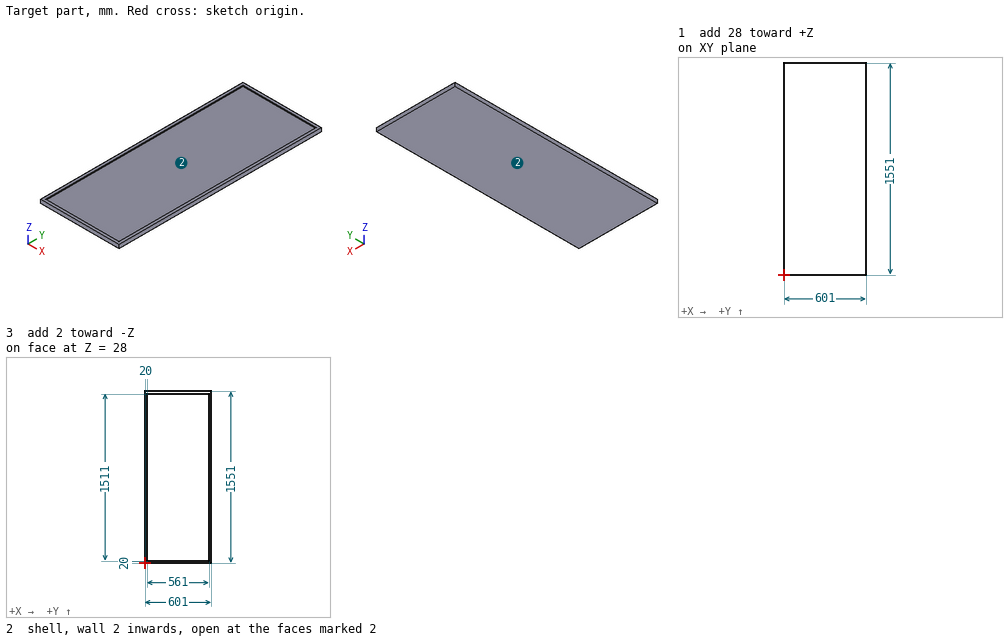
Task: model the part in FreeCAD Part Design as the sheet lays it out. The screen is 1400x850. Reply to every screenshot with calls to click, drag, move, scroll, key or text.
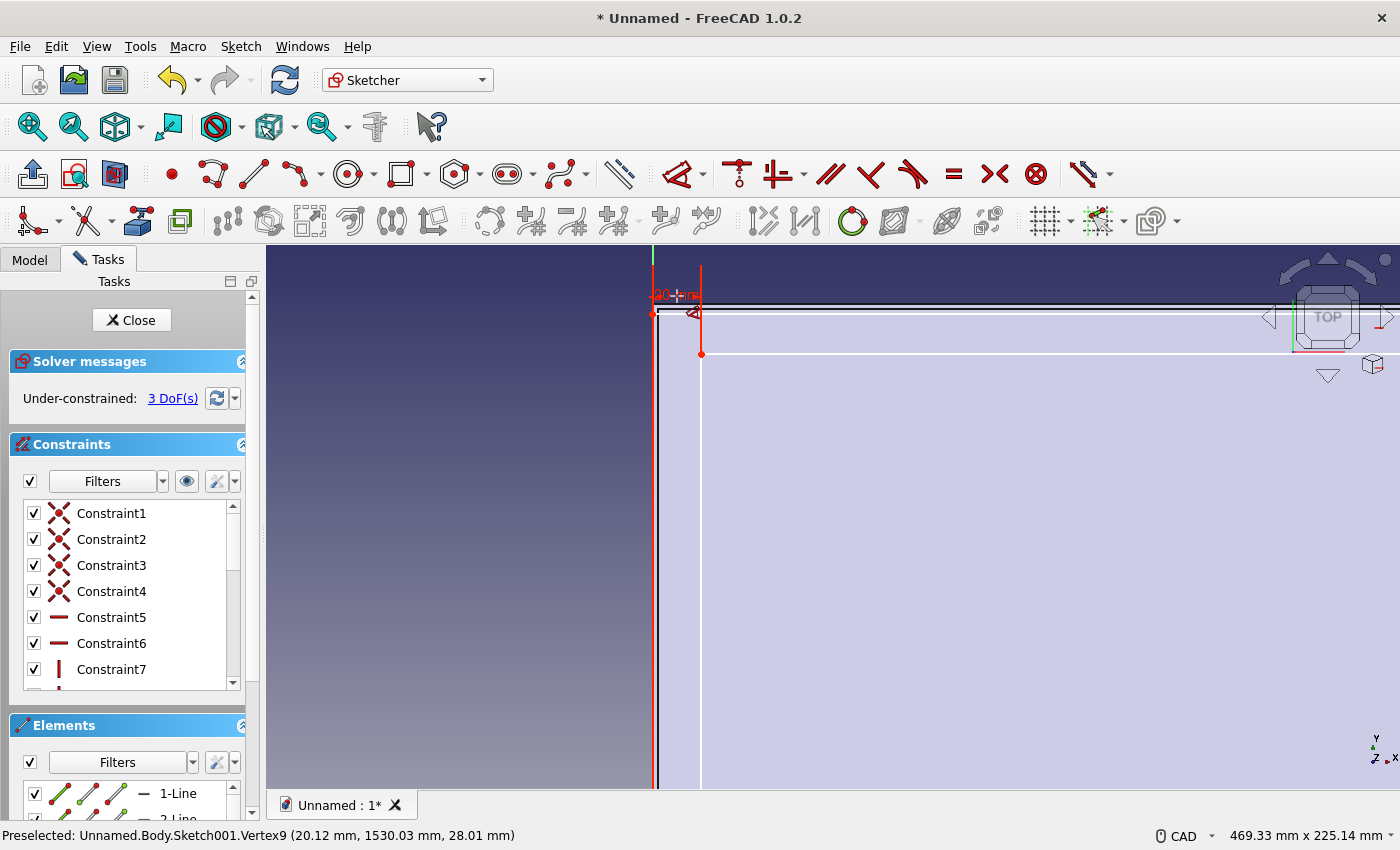
scroll(703, 351, down, 12)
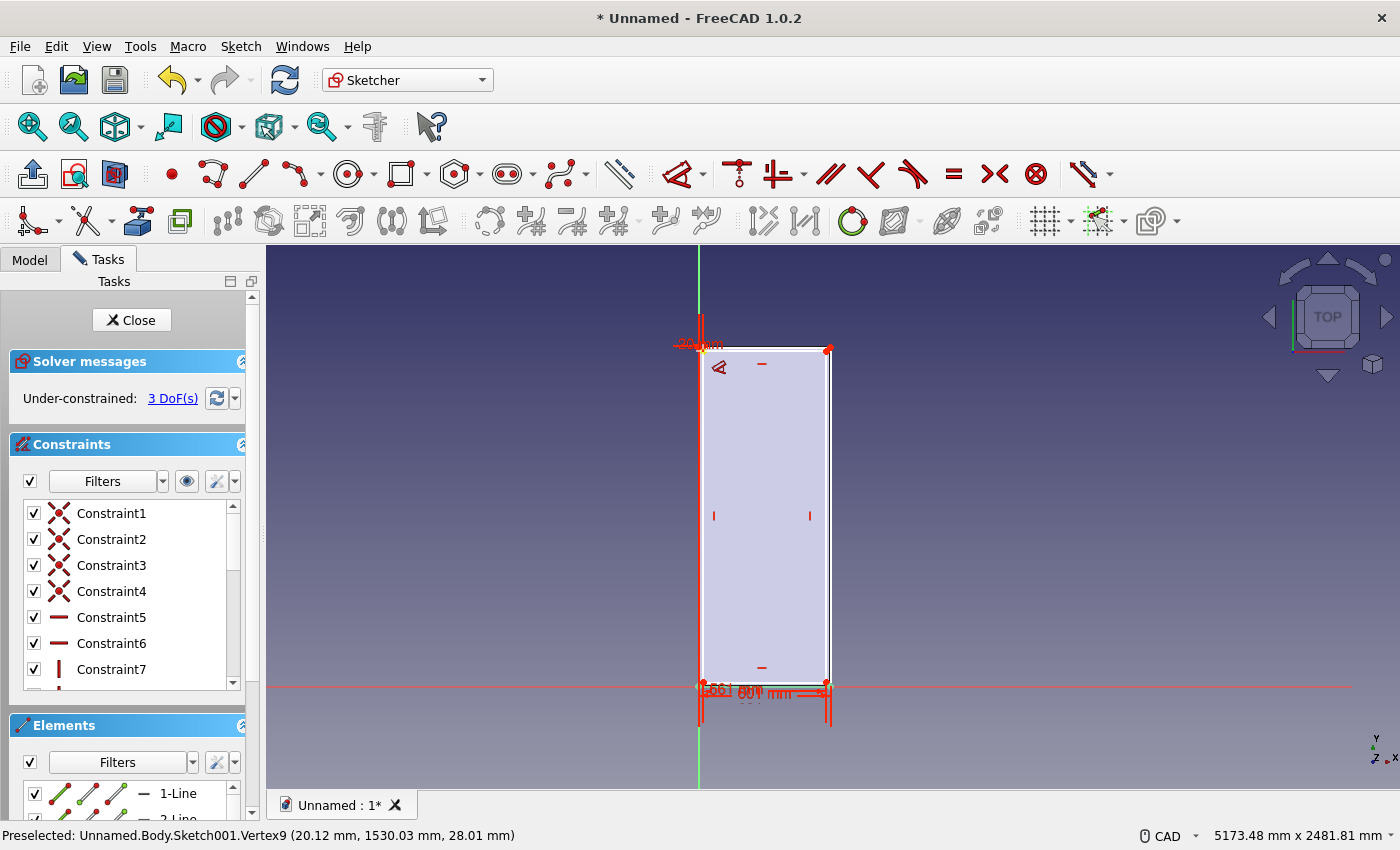
scroll(703, 683, up, 12)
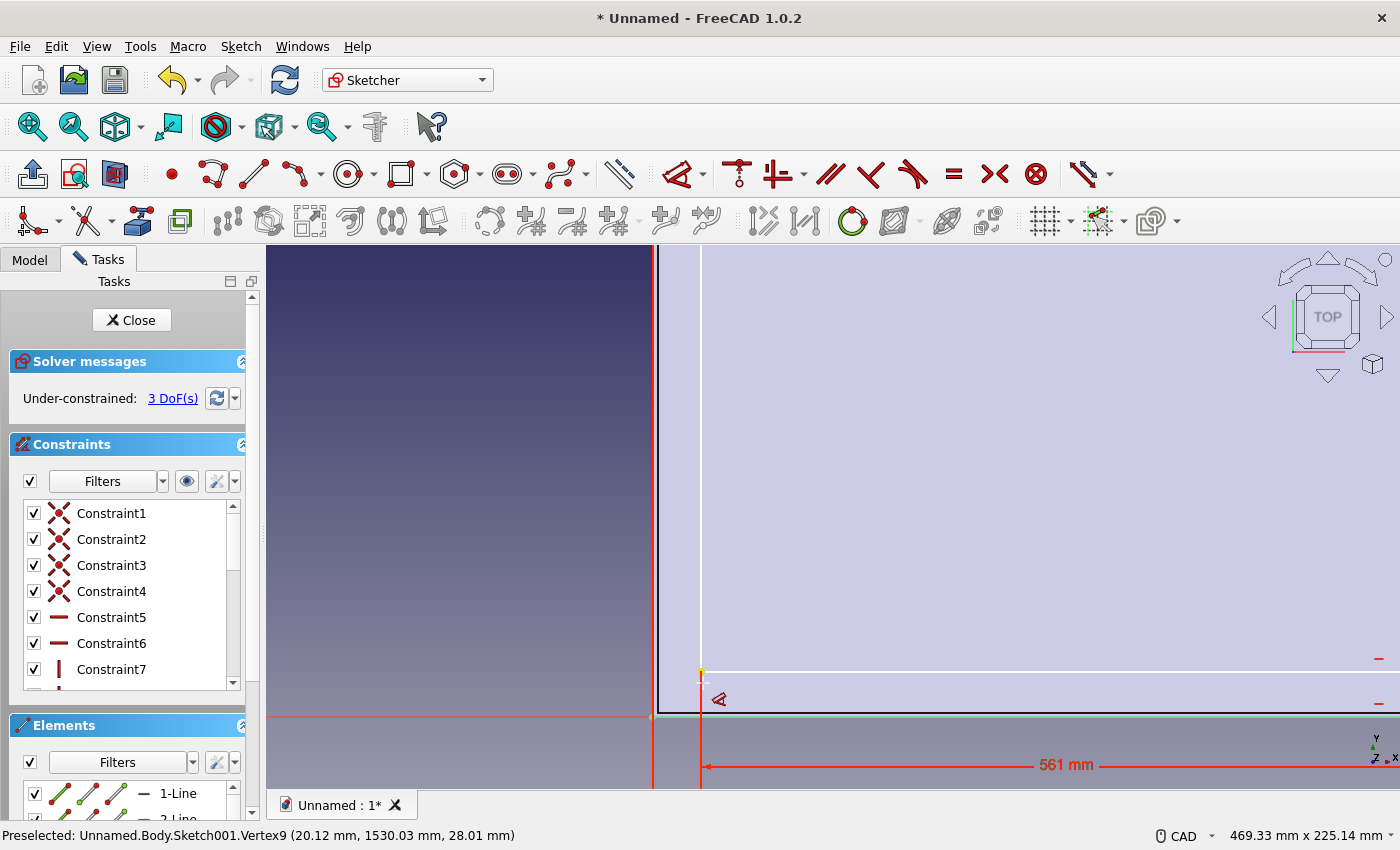
click(701, 672)
click(619, 695)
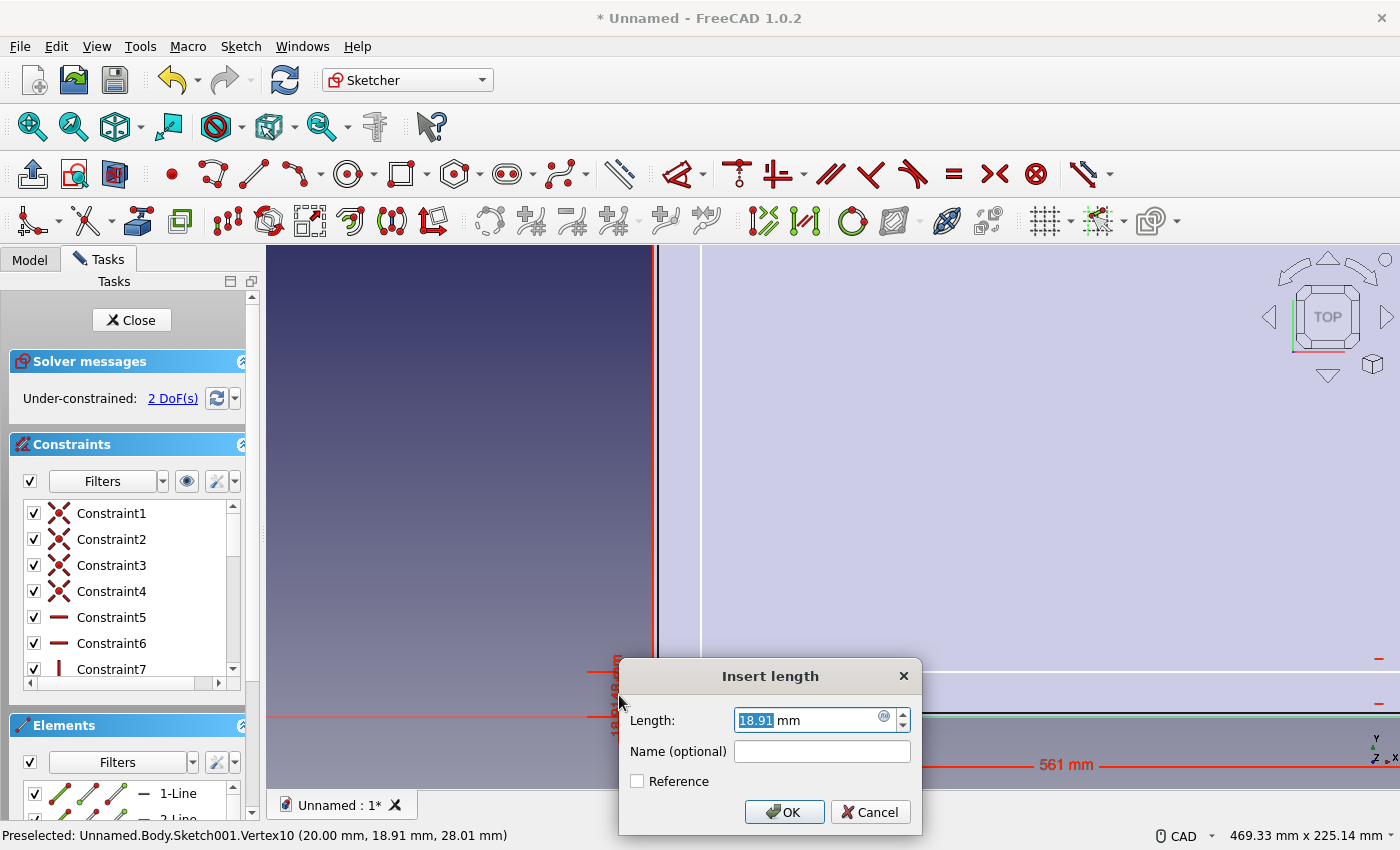
text(20)
key(Return)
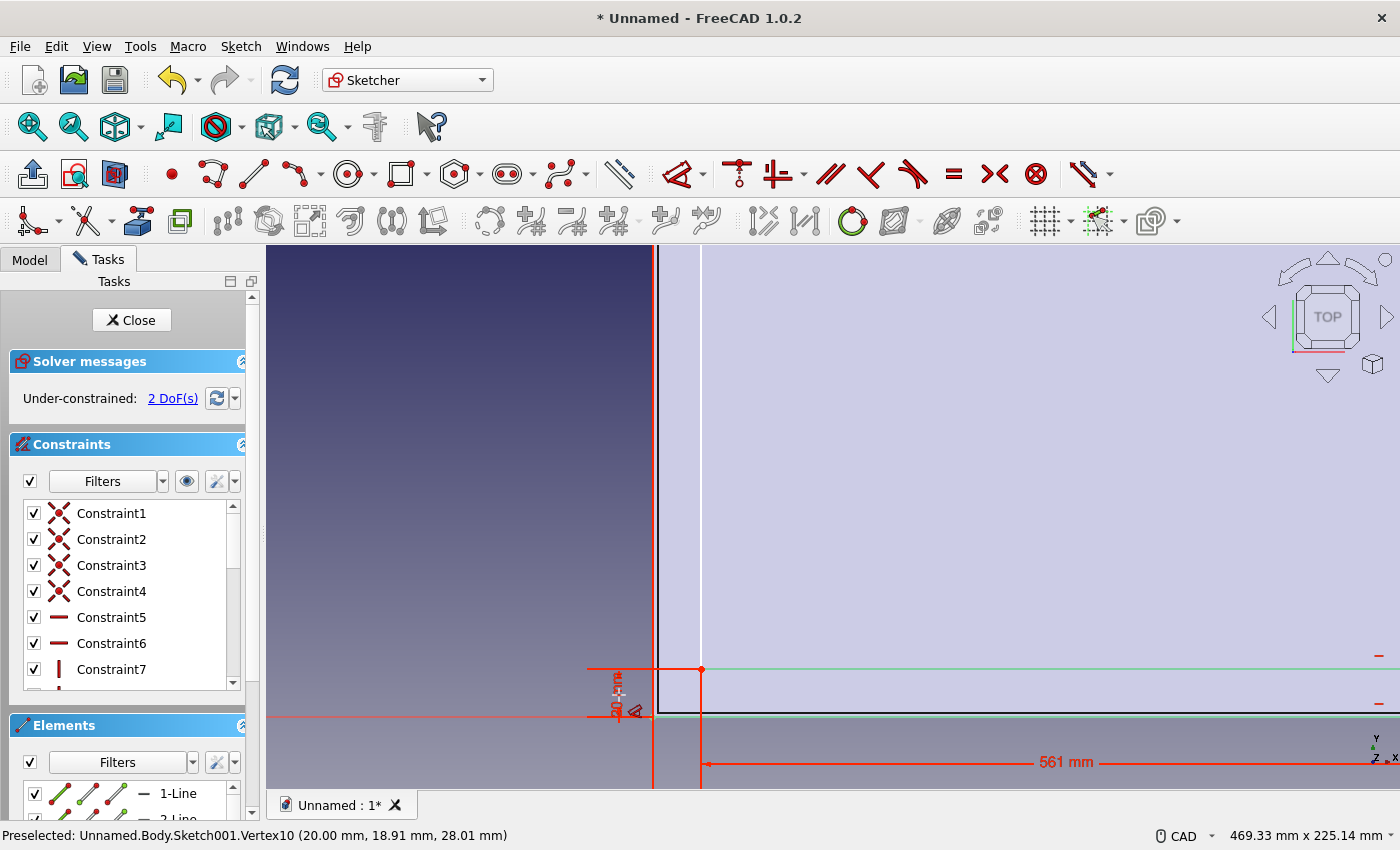
scroll(703, 684, down, 12)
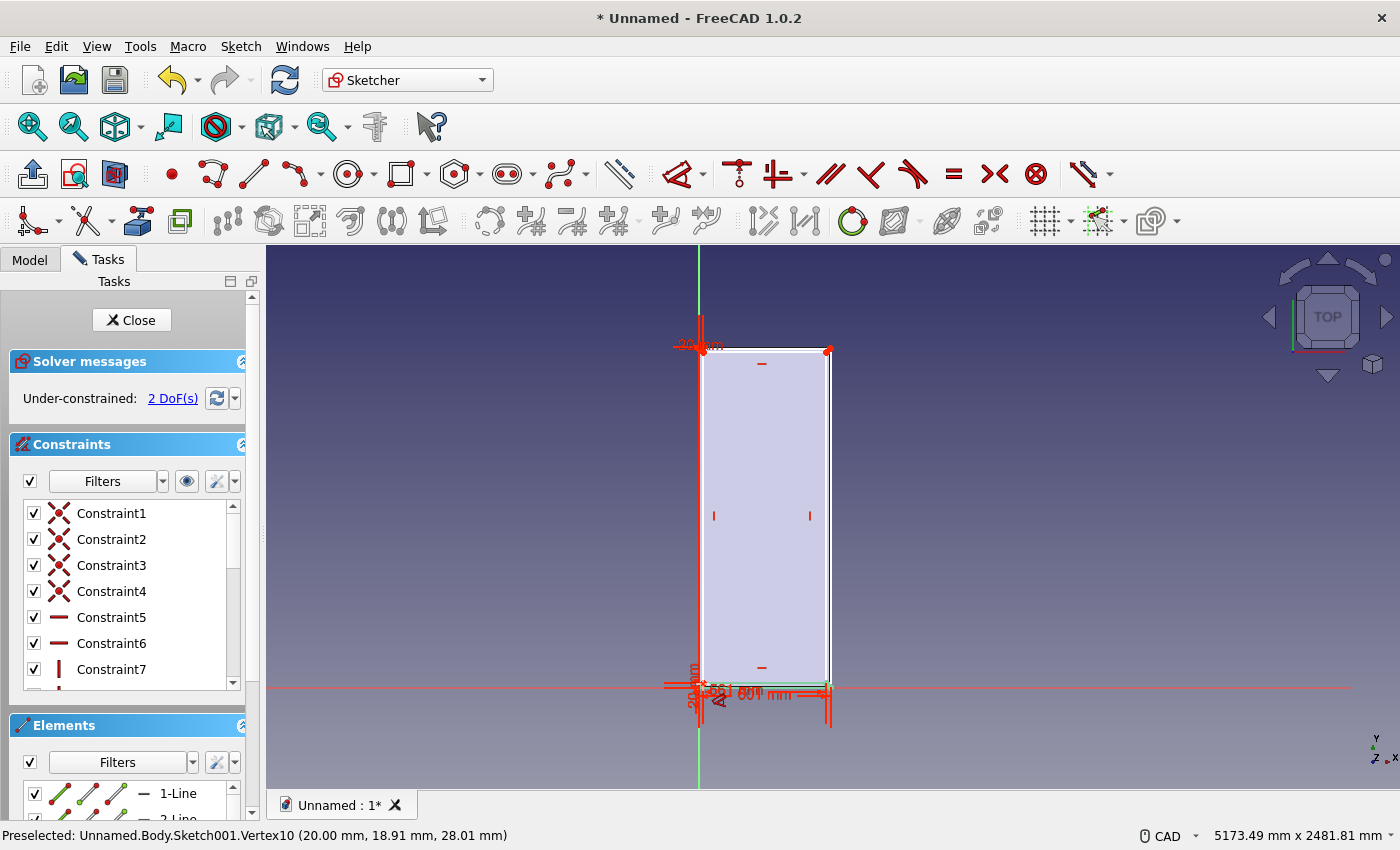
scroll(831, 586, up, 6)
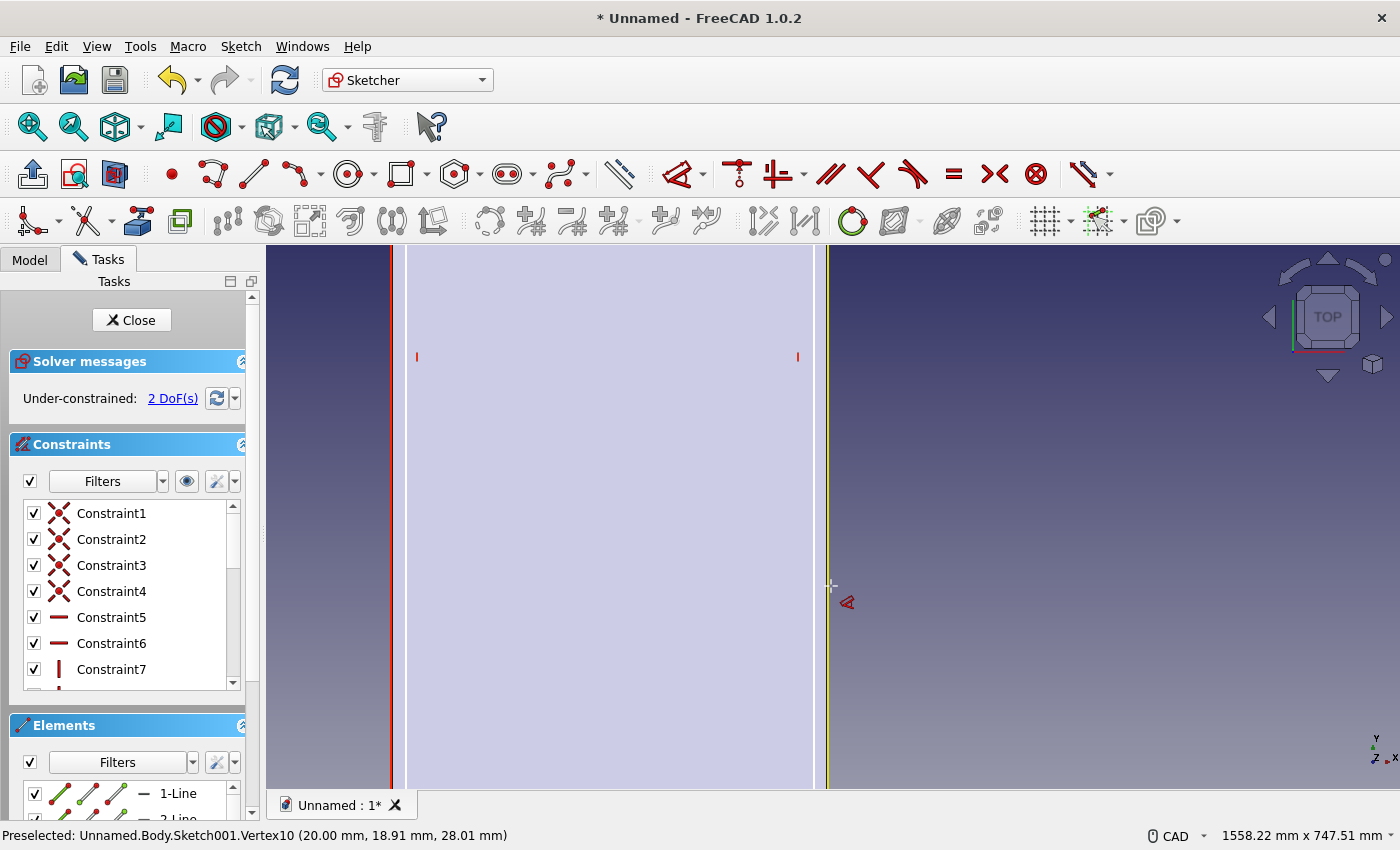
click(828, 585)
click(862, 517)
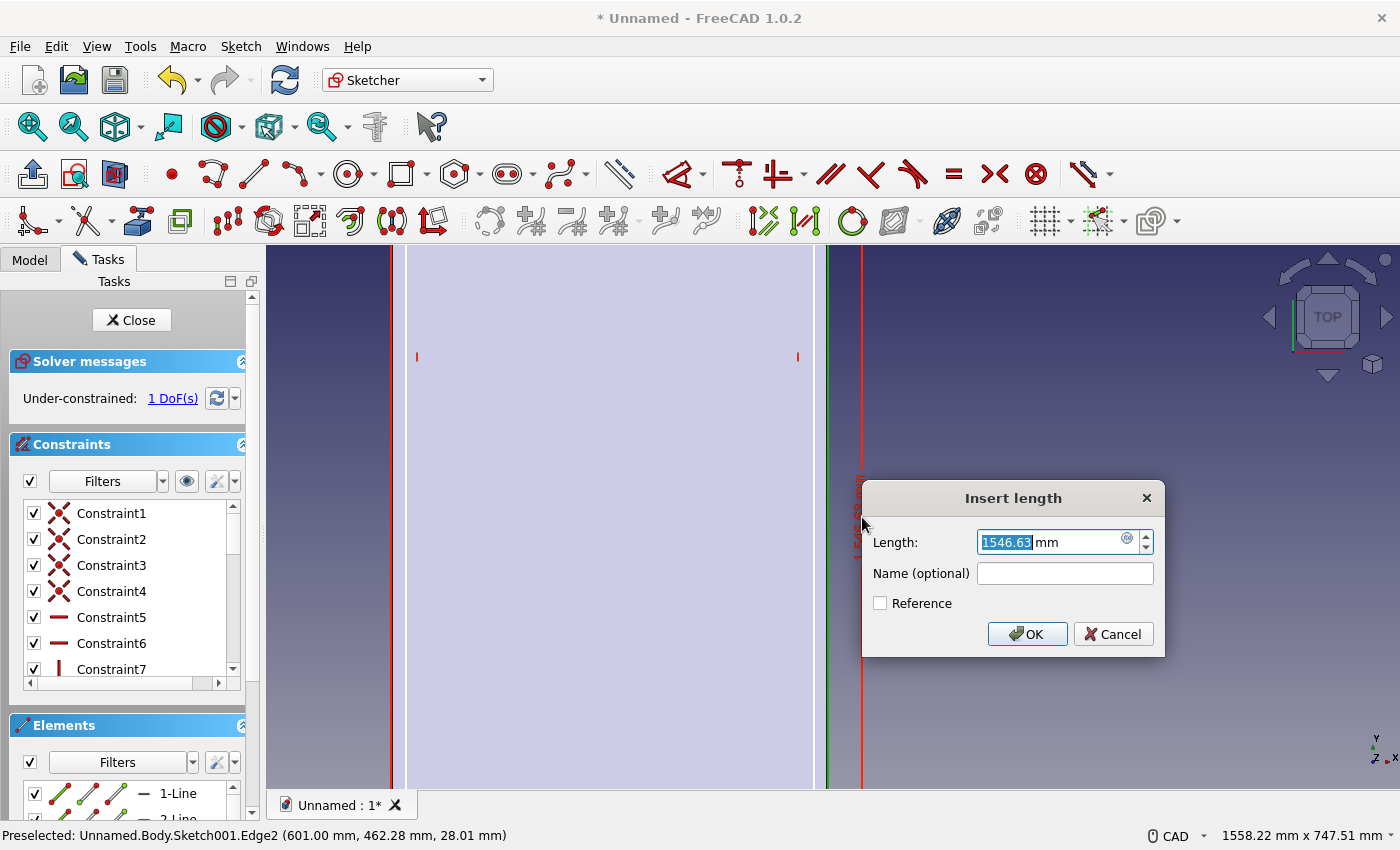
text(1551)
key(Return)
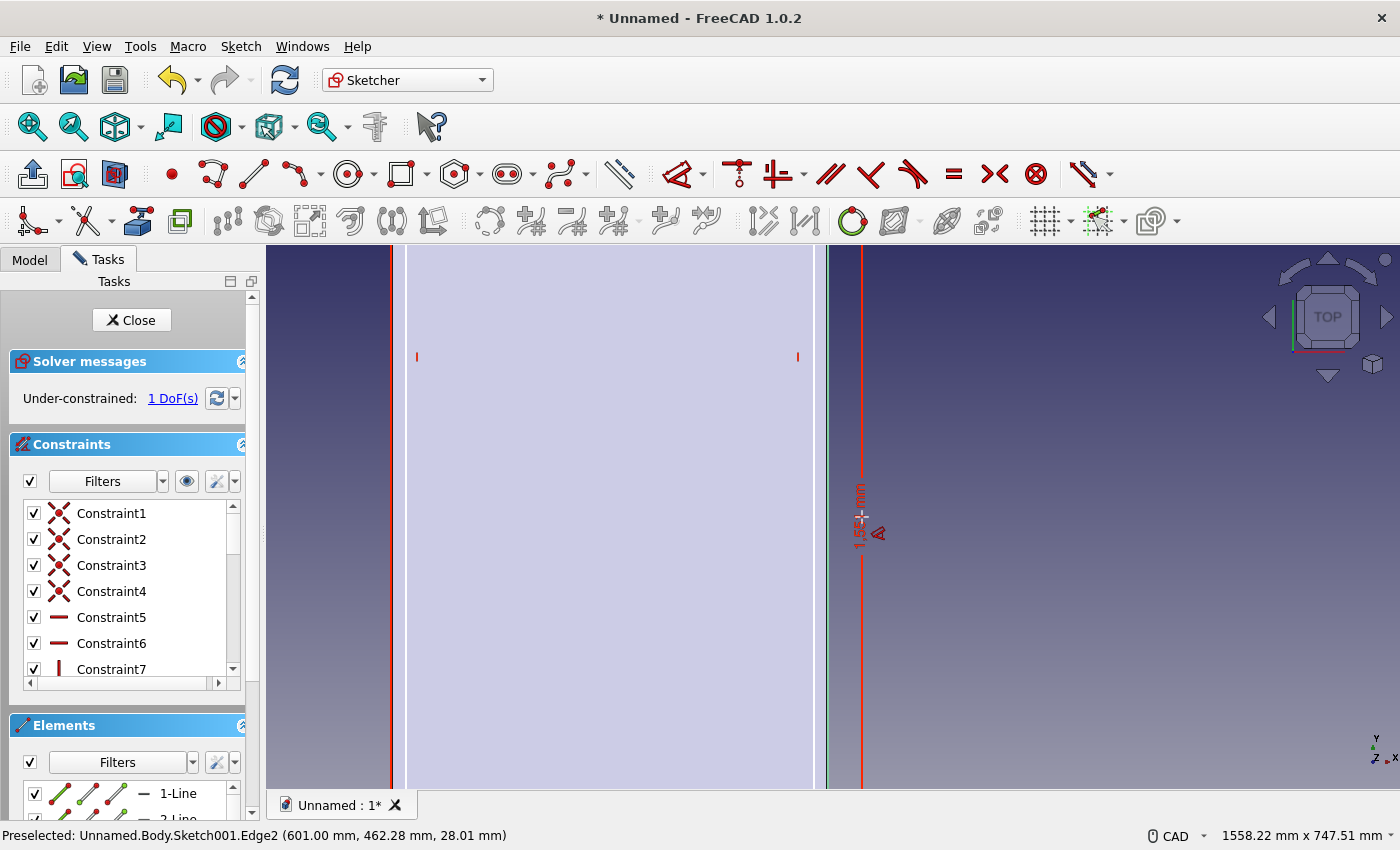
click(406, 578)
click(372, 517)